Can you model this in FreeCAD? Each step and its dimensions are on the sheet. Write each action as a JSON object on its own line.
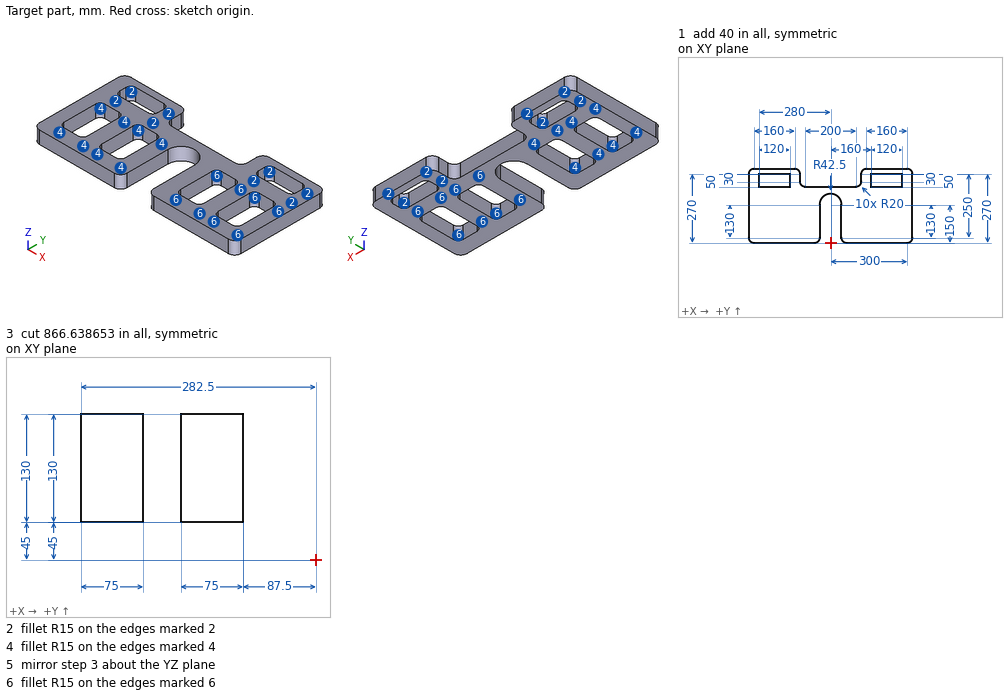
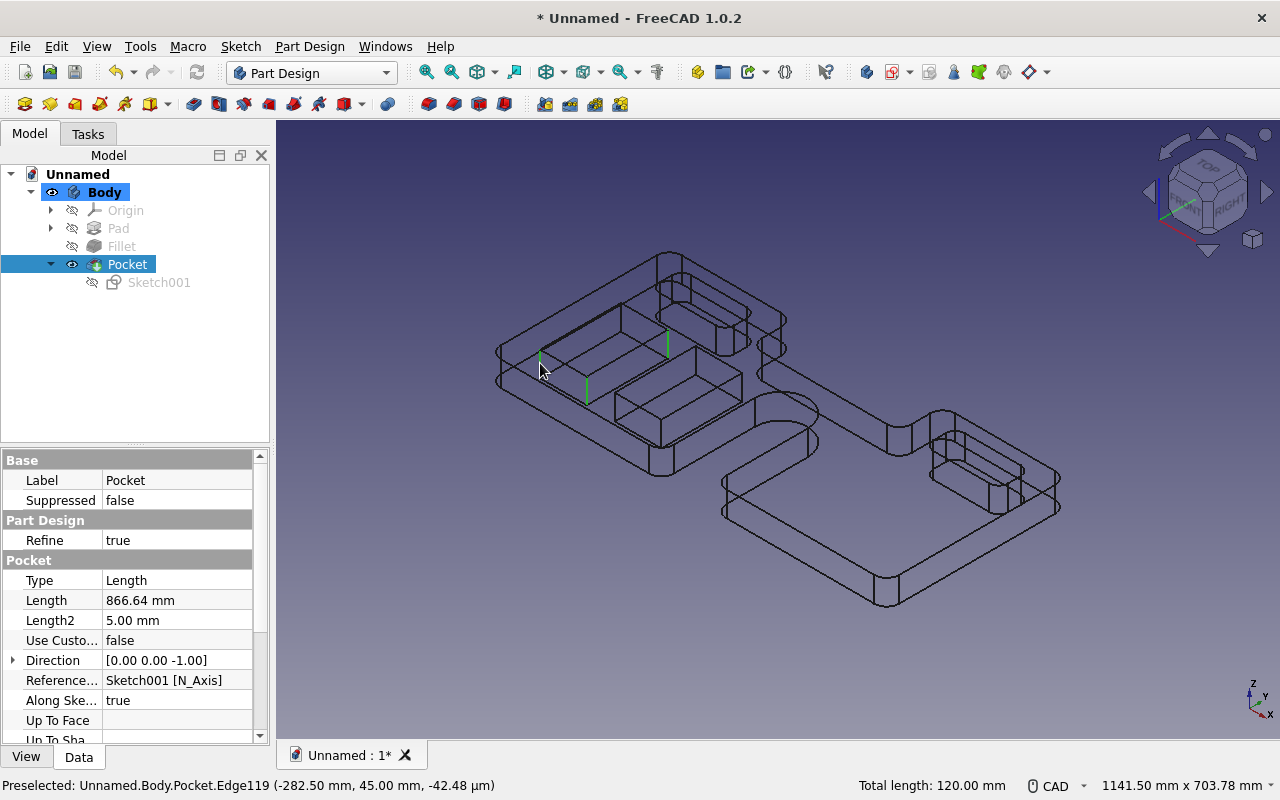
{"action": "left_click", "coordinate": [621, 316], "text": "ctrl"}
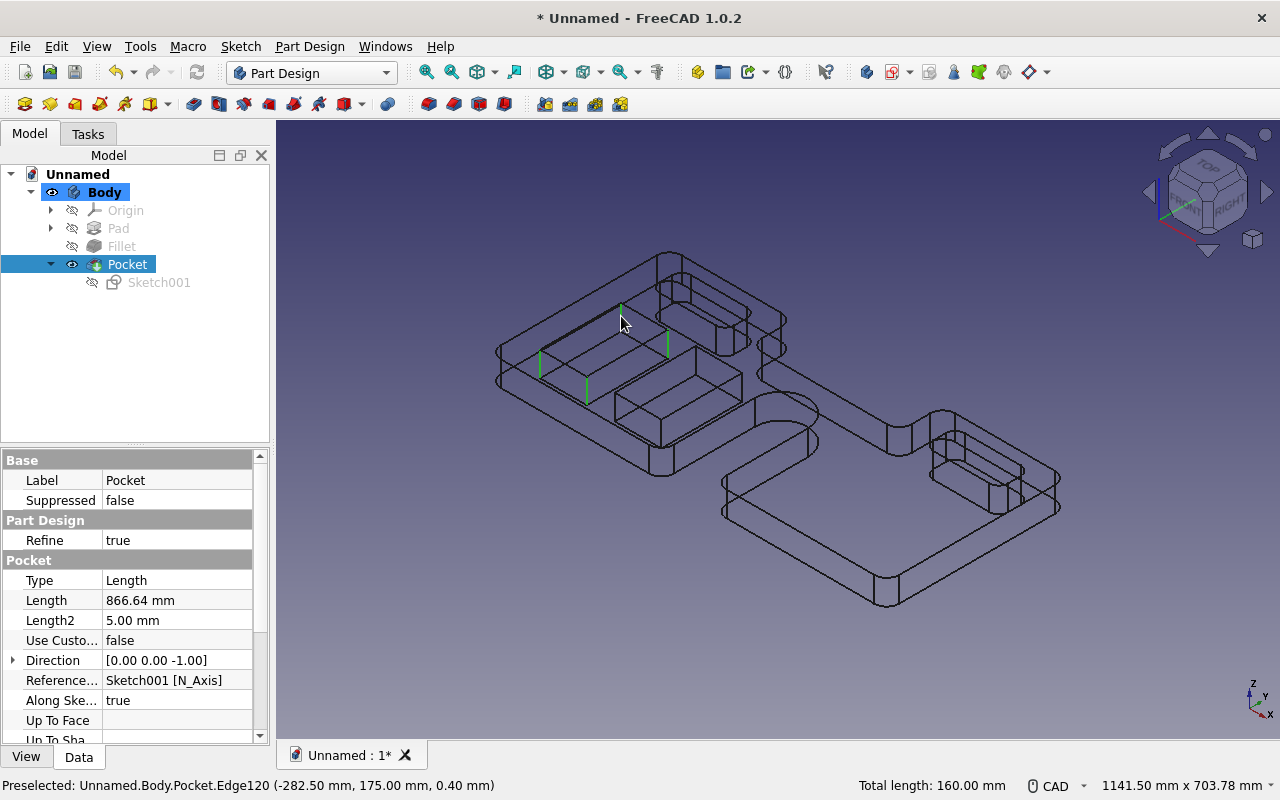
{"action": "left_click", "coordinate": [742, 386], "text": "ctrl"}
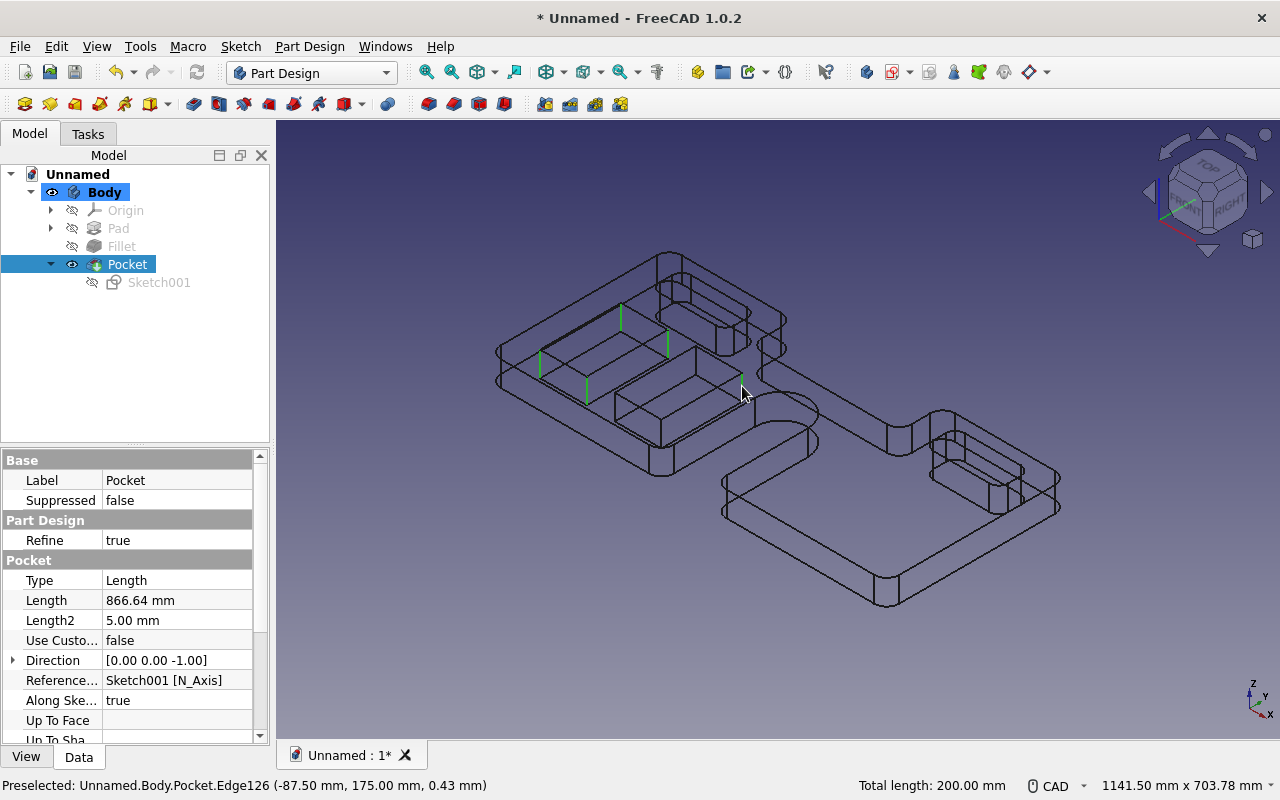
{"action": "left_click", "coordinate": [661, 433], "text": "ctrl"}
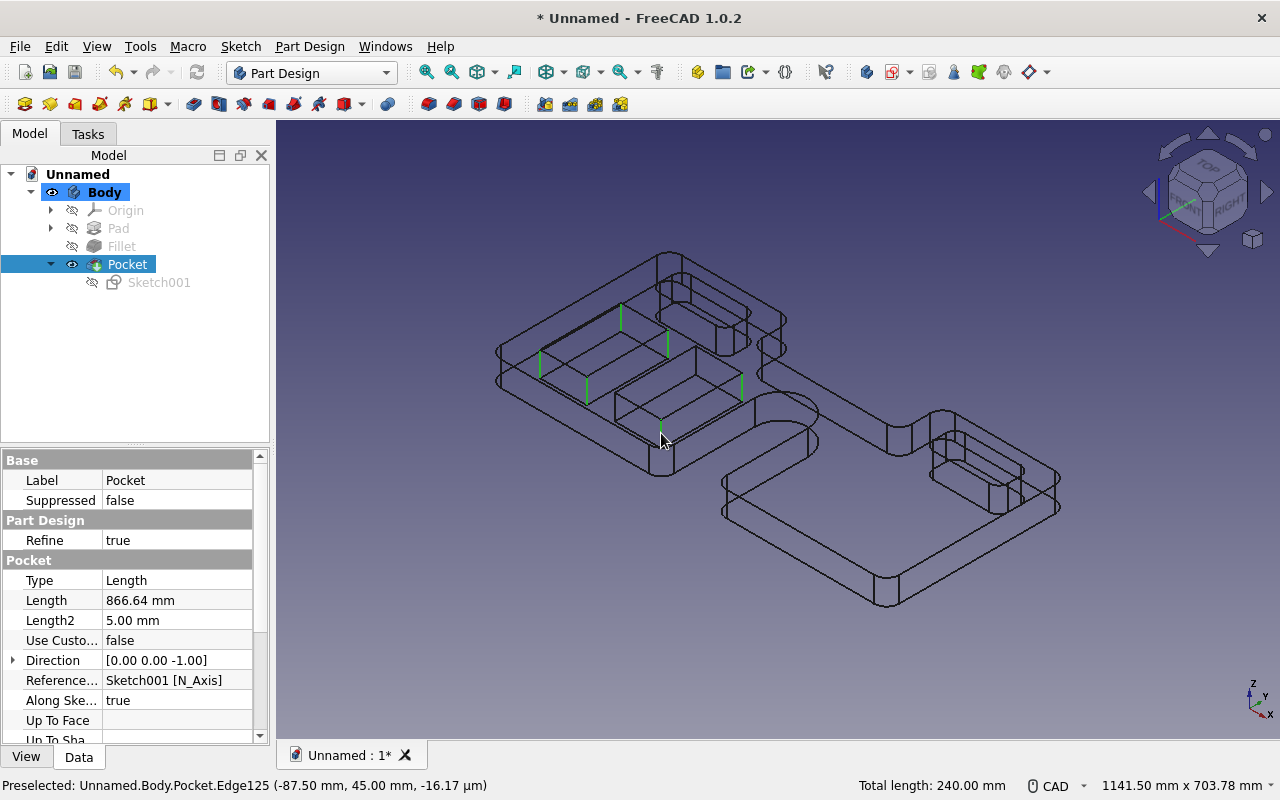
{"action": "left_click", "coordinate": [615, 406], "text": "ctrl"}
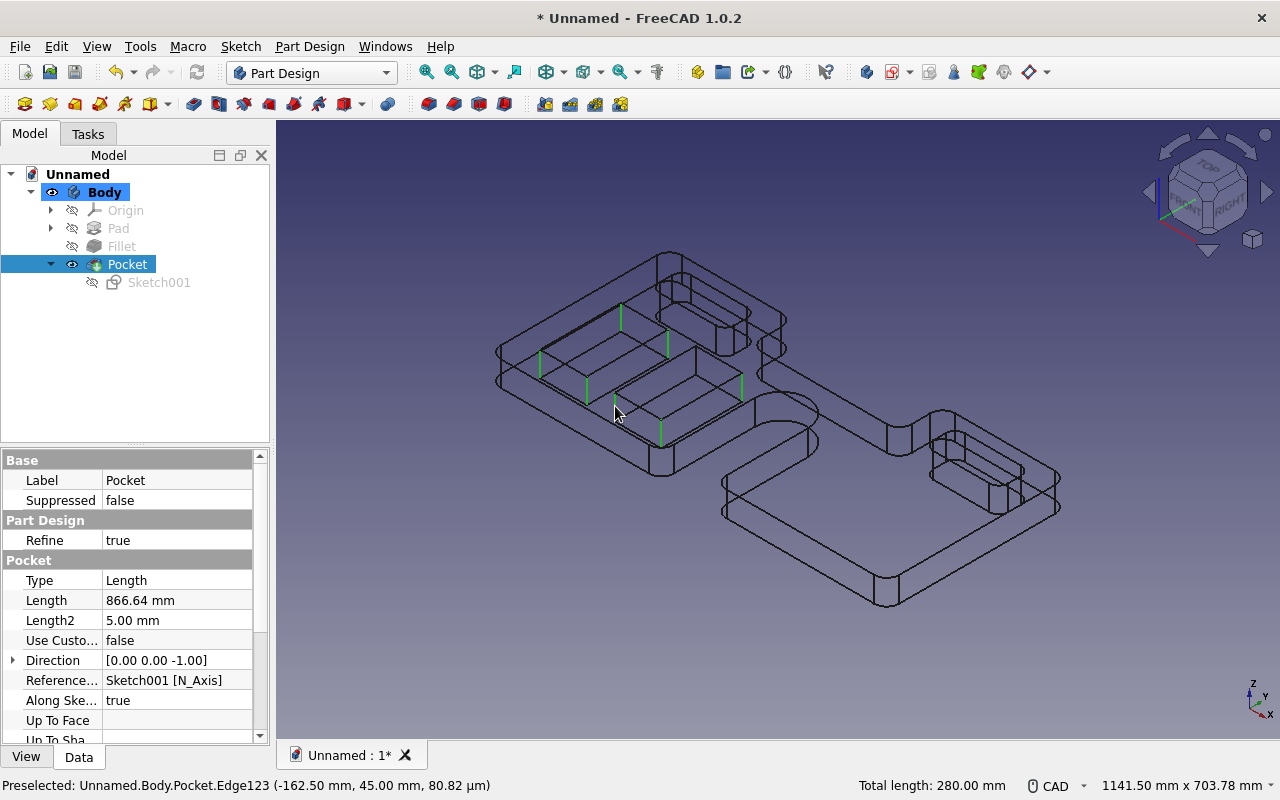
{"action": "left_click", "coordinate": [696, 359], "text": "ctrl"}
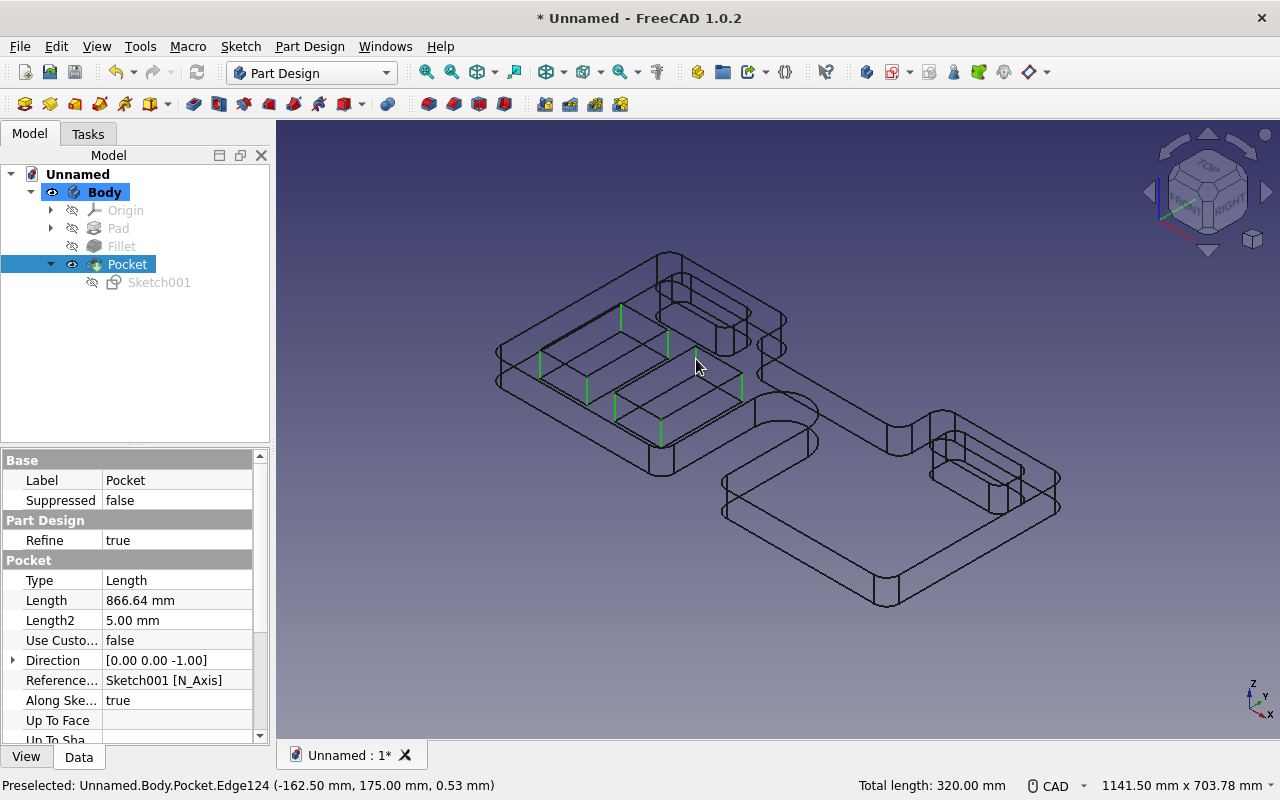
{"action": "key", "text": "v 1"}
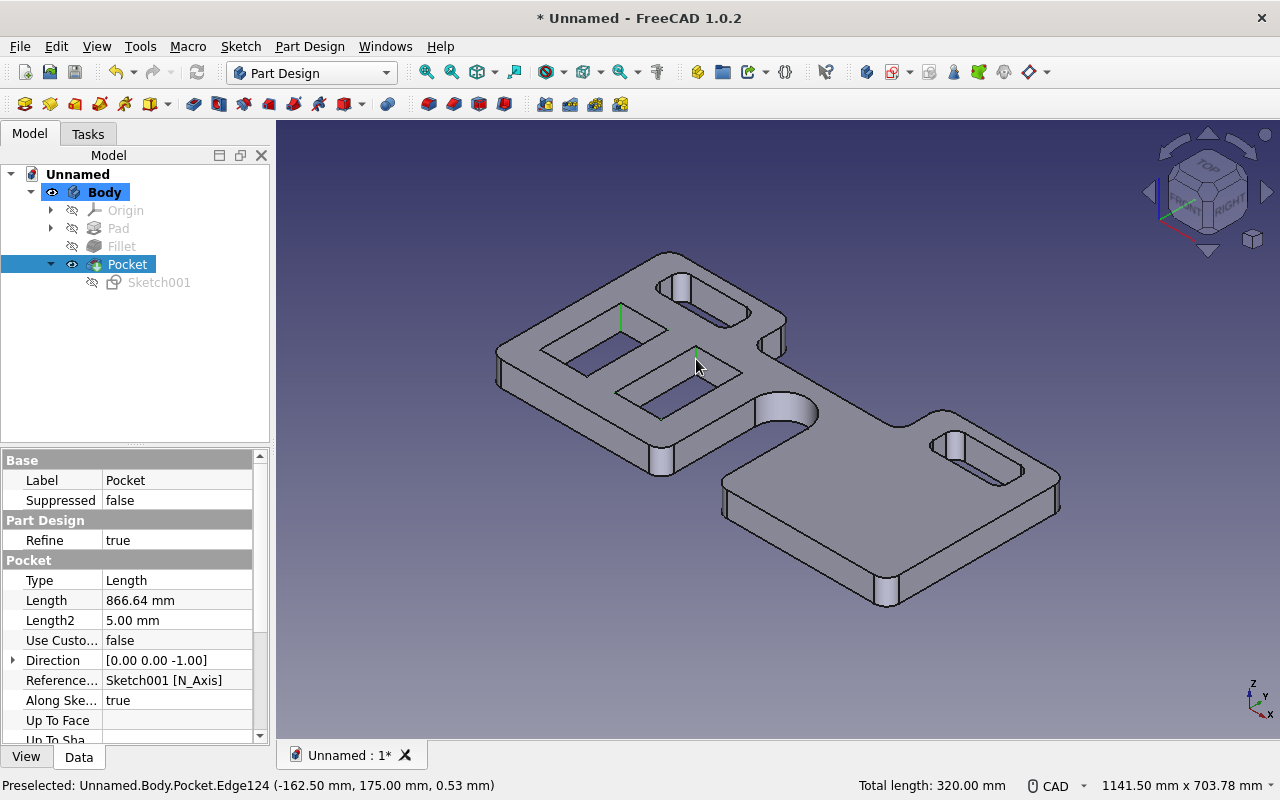
{"action": "left_click", "coordinate": [429, 104]}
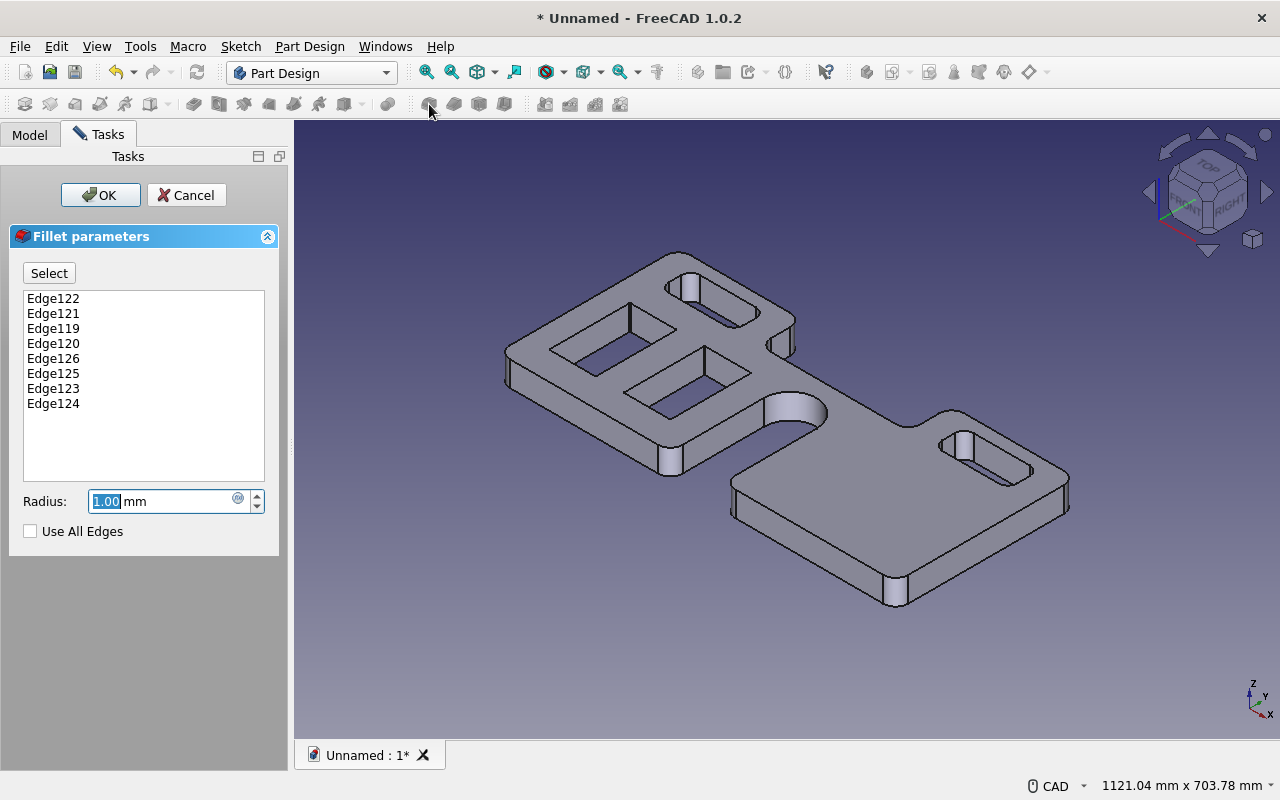
{"action": "type", "text": "15"}
{"action": "key", "text": "Tab"}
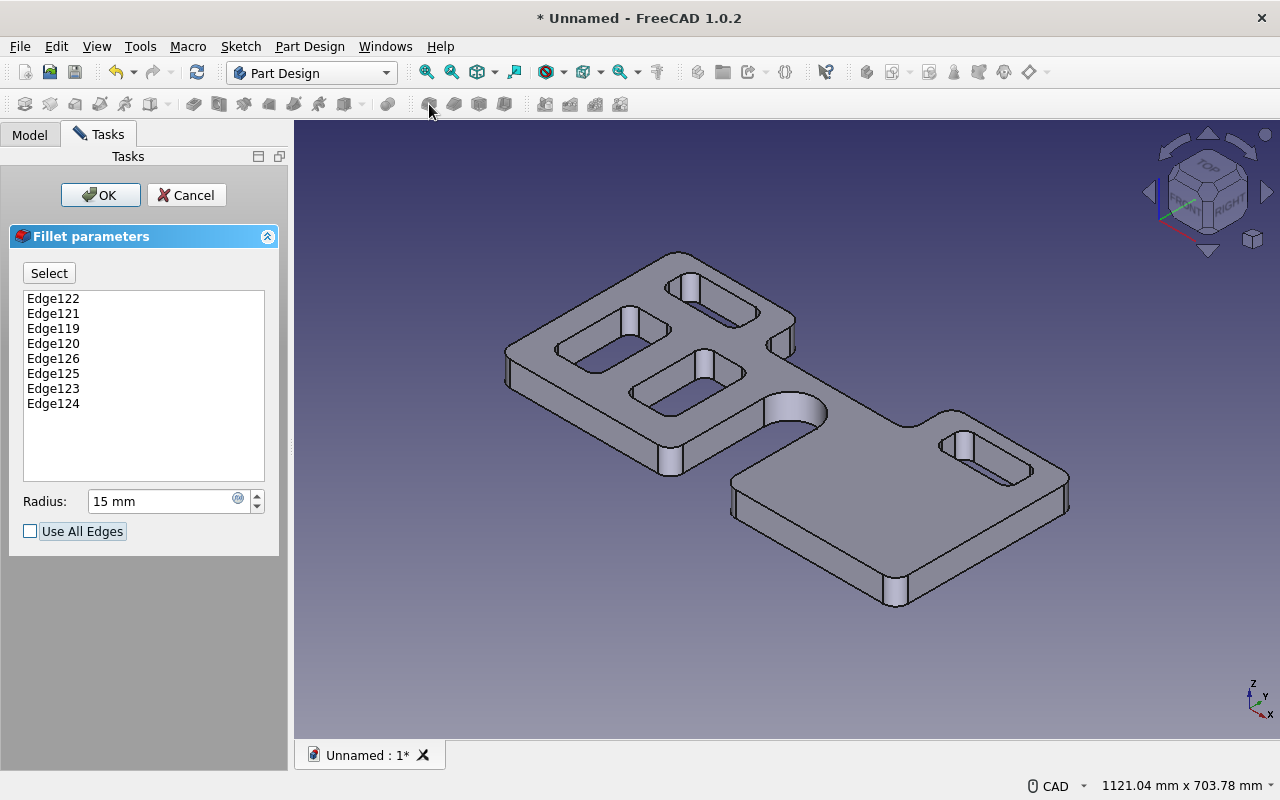
{"action": "left_click", "coordinate": [101, 195]}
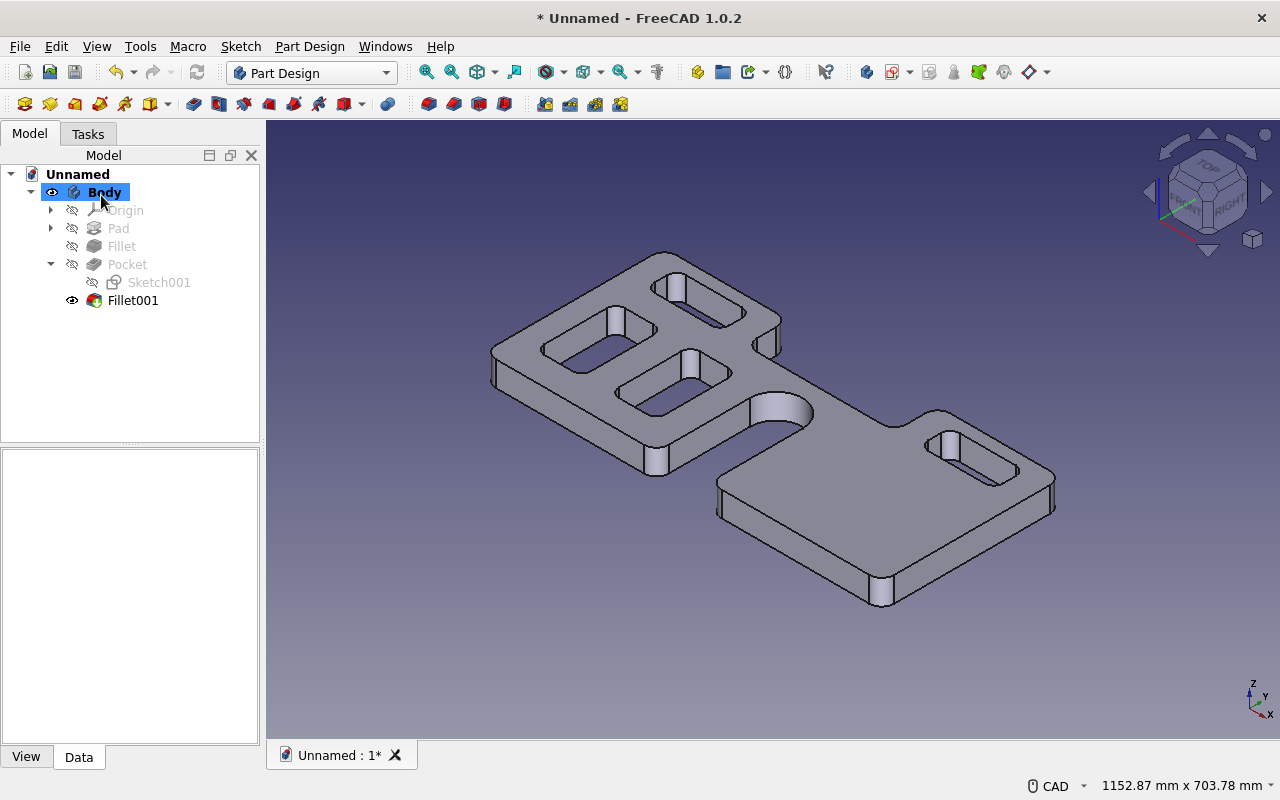
{"action": "left_click", "coordinate": [117, 264]}